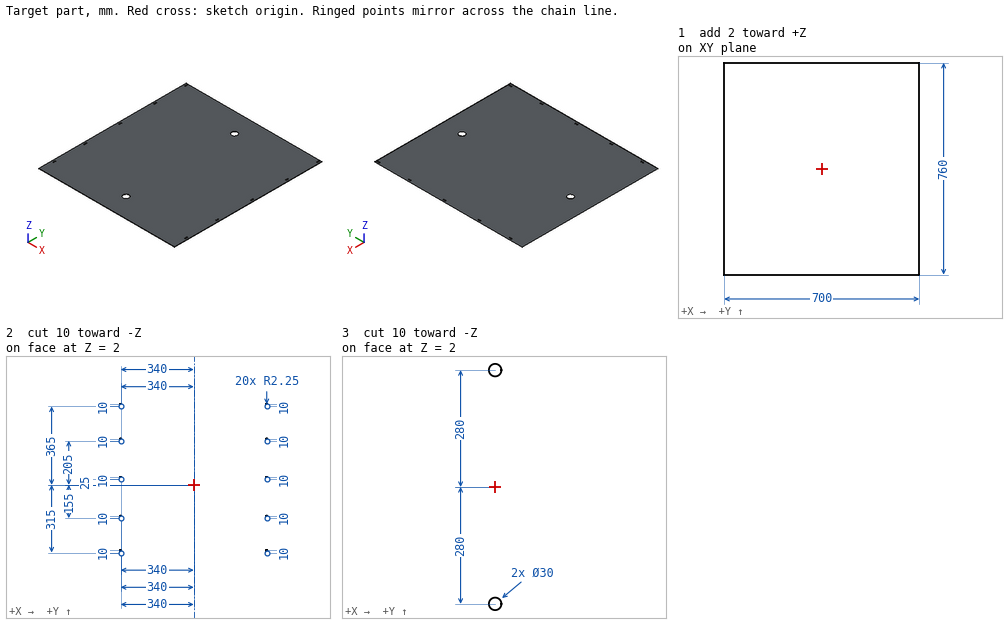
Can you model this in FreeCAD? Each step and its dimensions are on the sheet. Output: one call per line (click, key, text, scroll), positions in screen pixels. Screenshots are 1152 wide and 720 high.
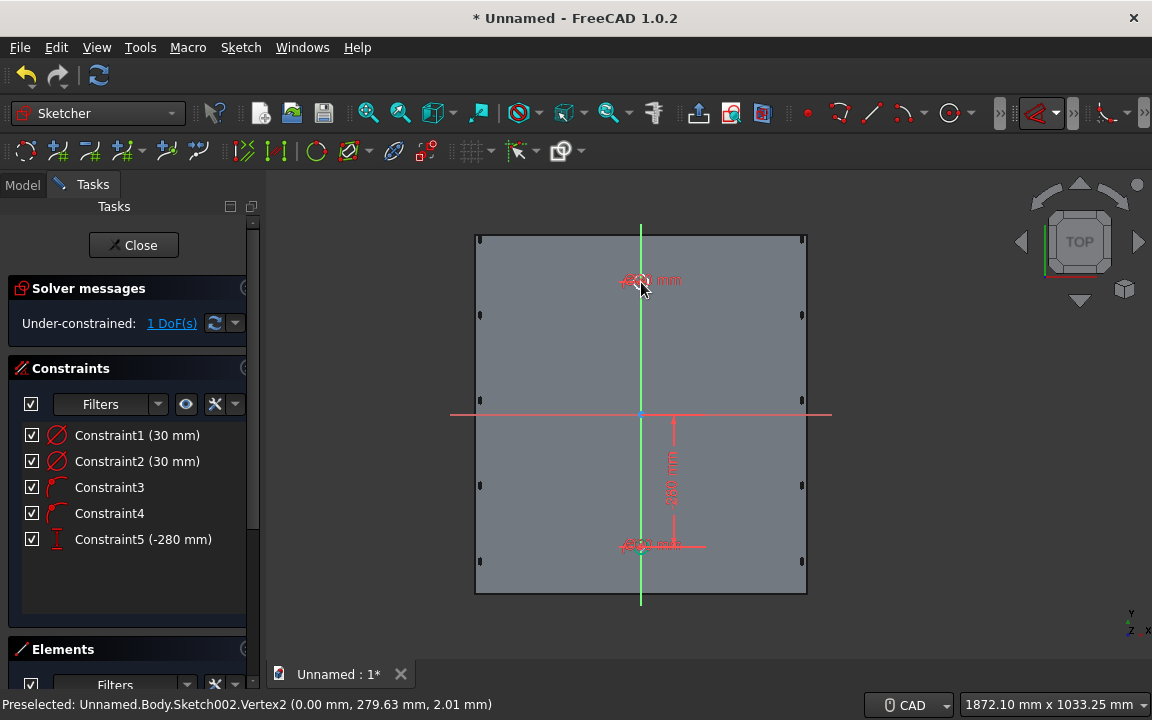
click(1058, 114)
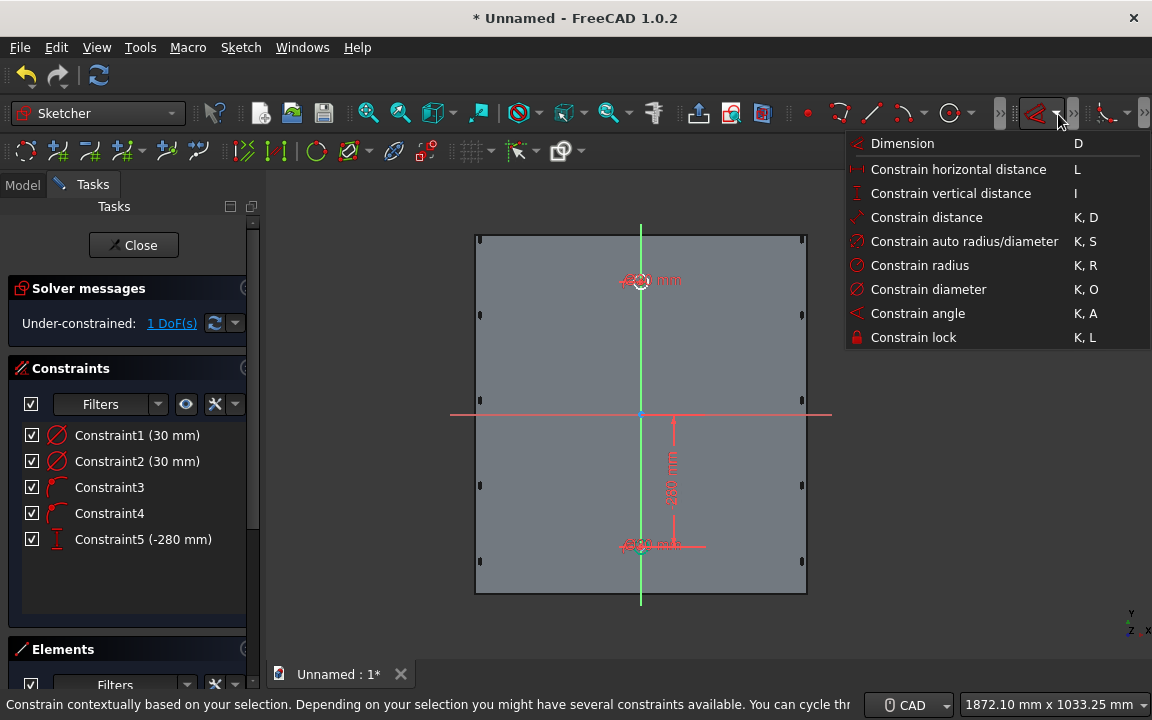
click(998, 193)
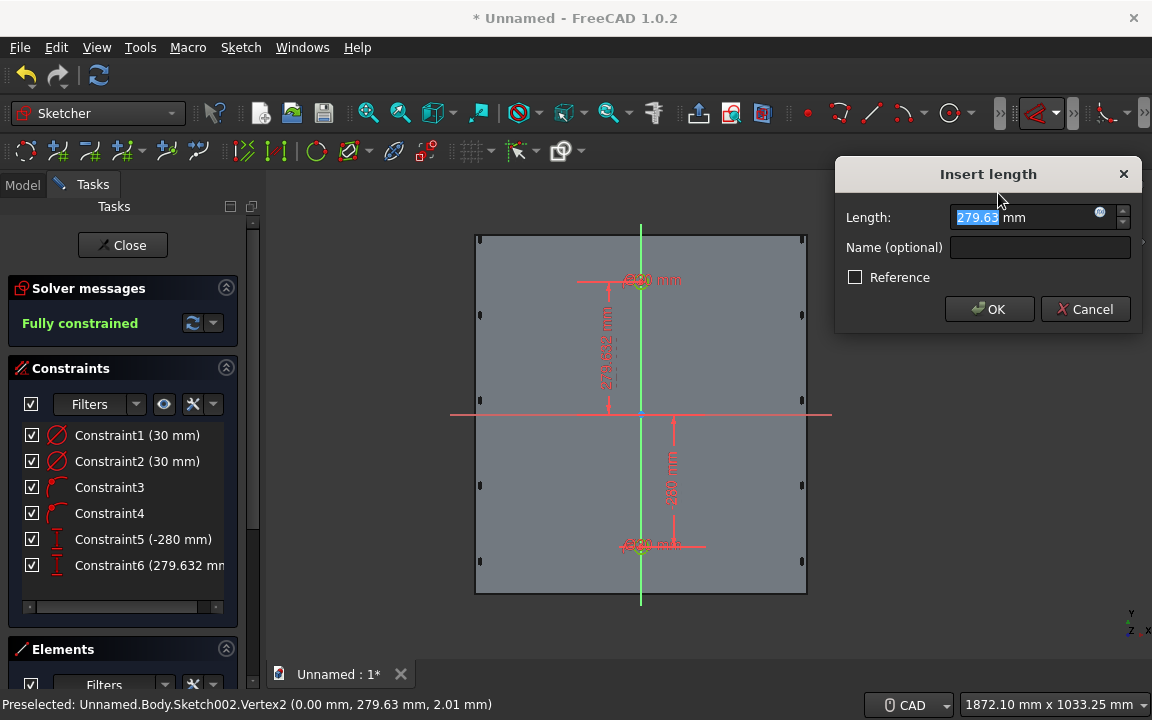
text(280)
key(Return)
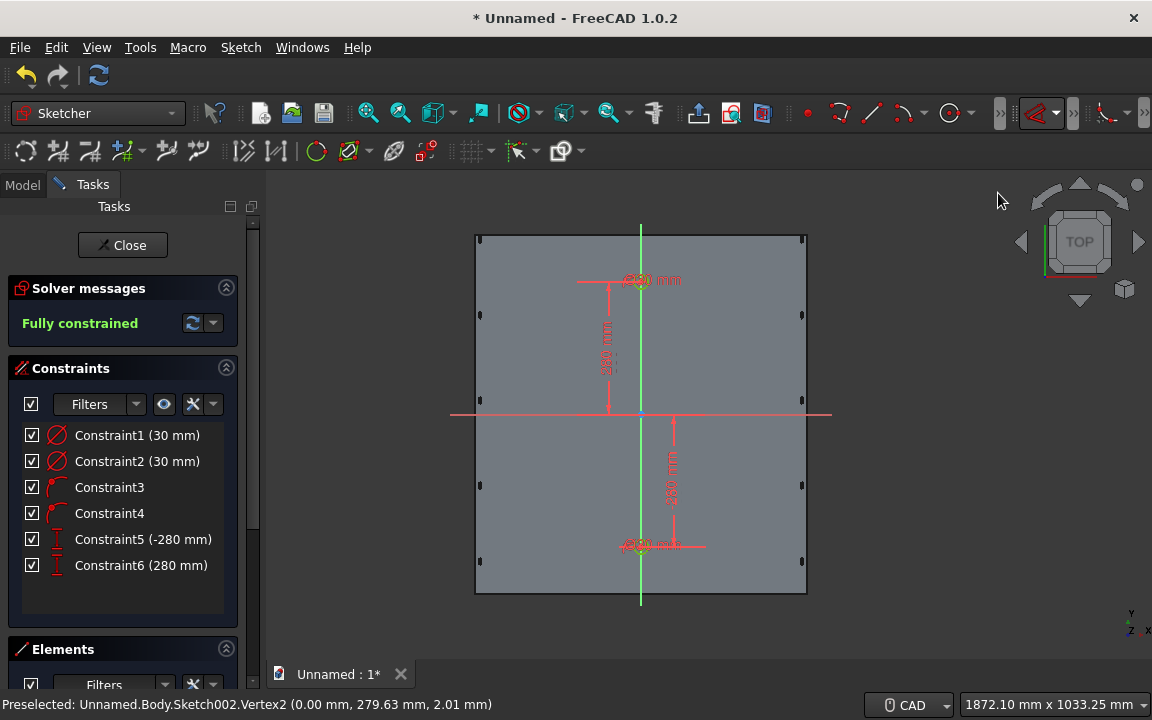
click(123, 245)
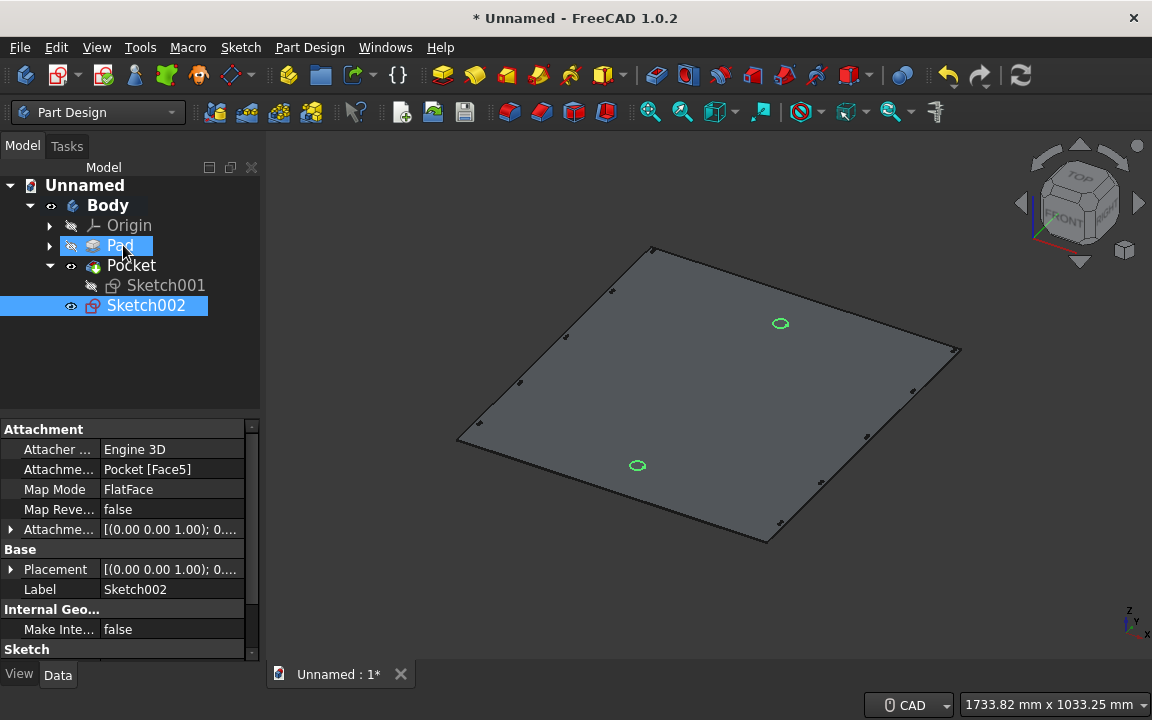
click(658, 76)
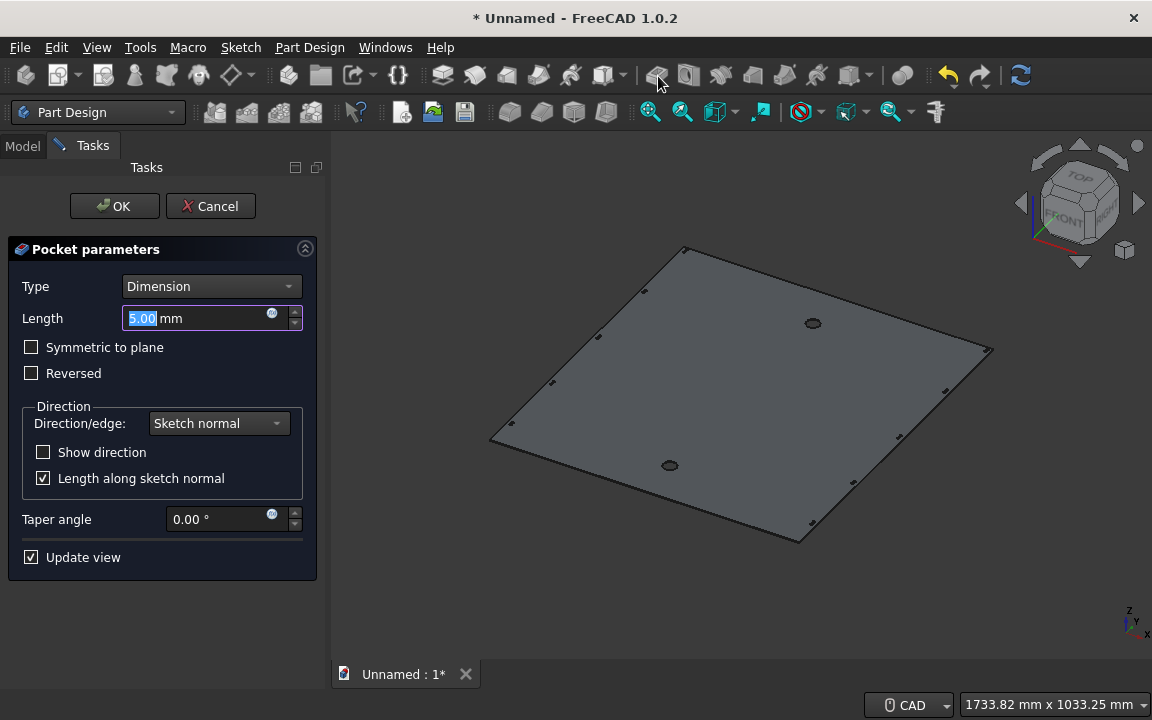
text(10)
key(Tab)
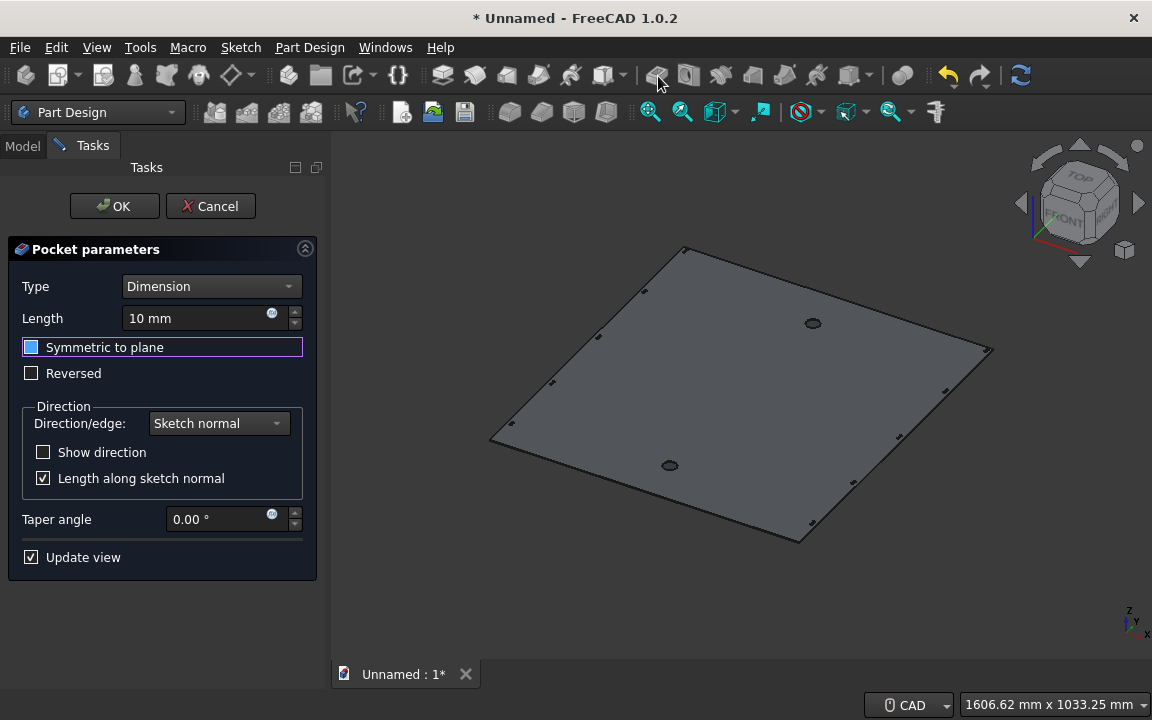
click(115, 206)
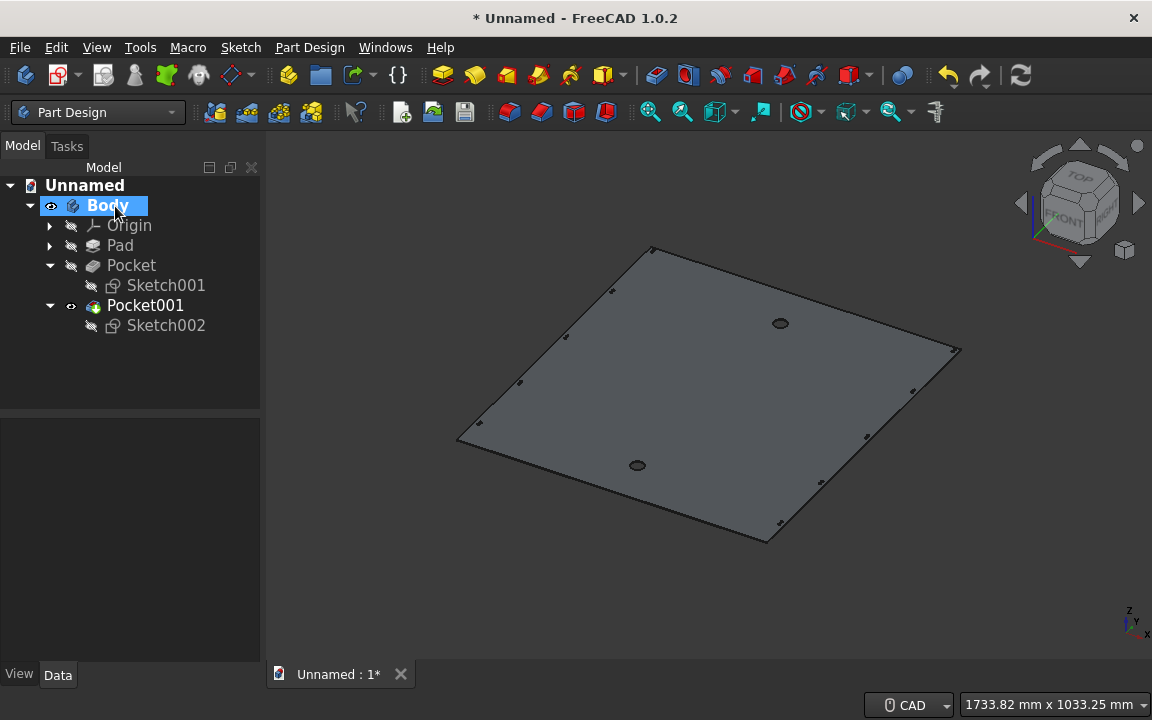
key(0)